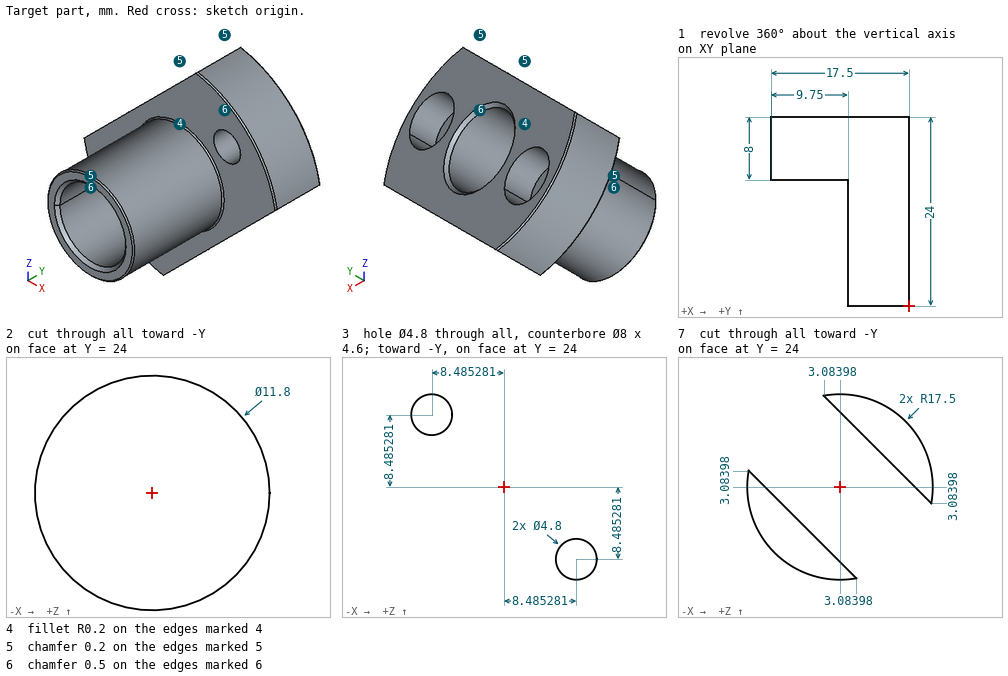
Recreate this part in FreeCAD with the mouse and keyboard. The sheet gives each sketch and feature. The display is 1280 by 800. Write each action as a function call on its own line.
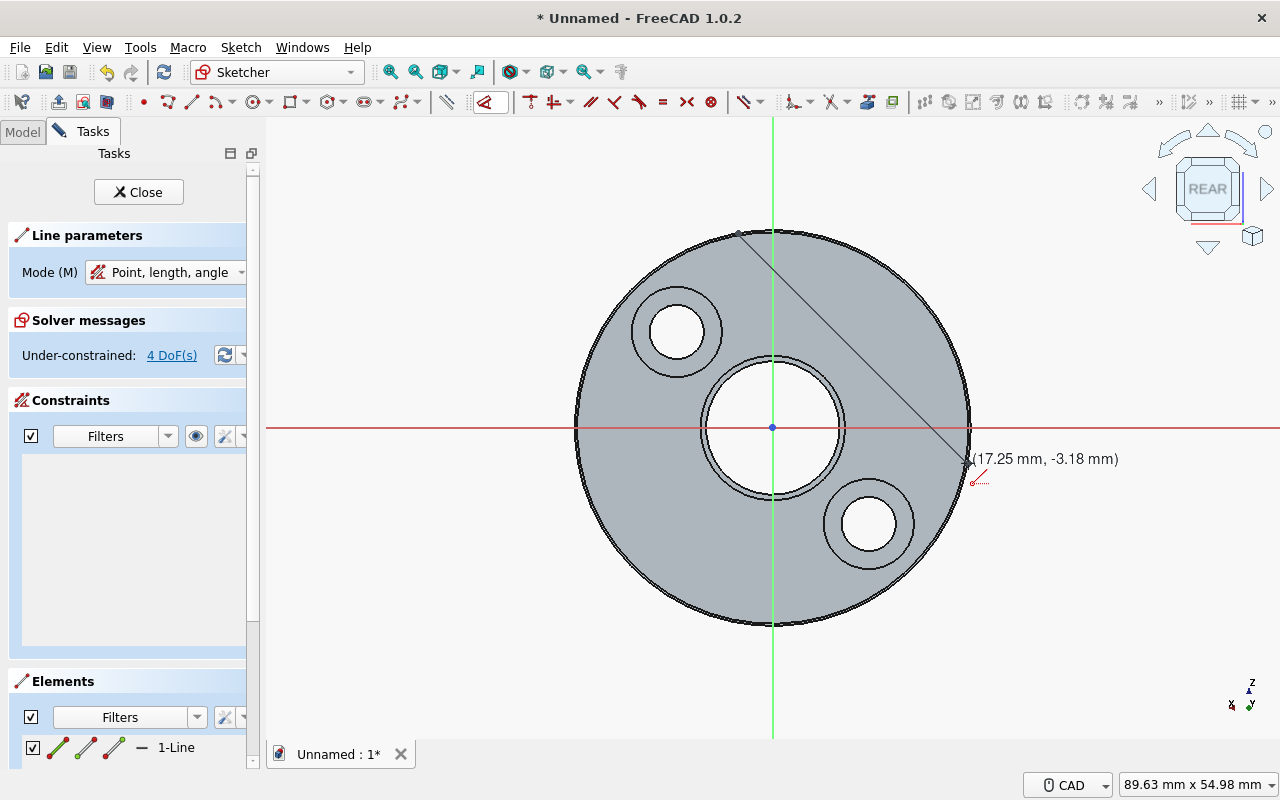
key(g)
key(3)
key(a)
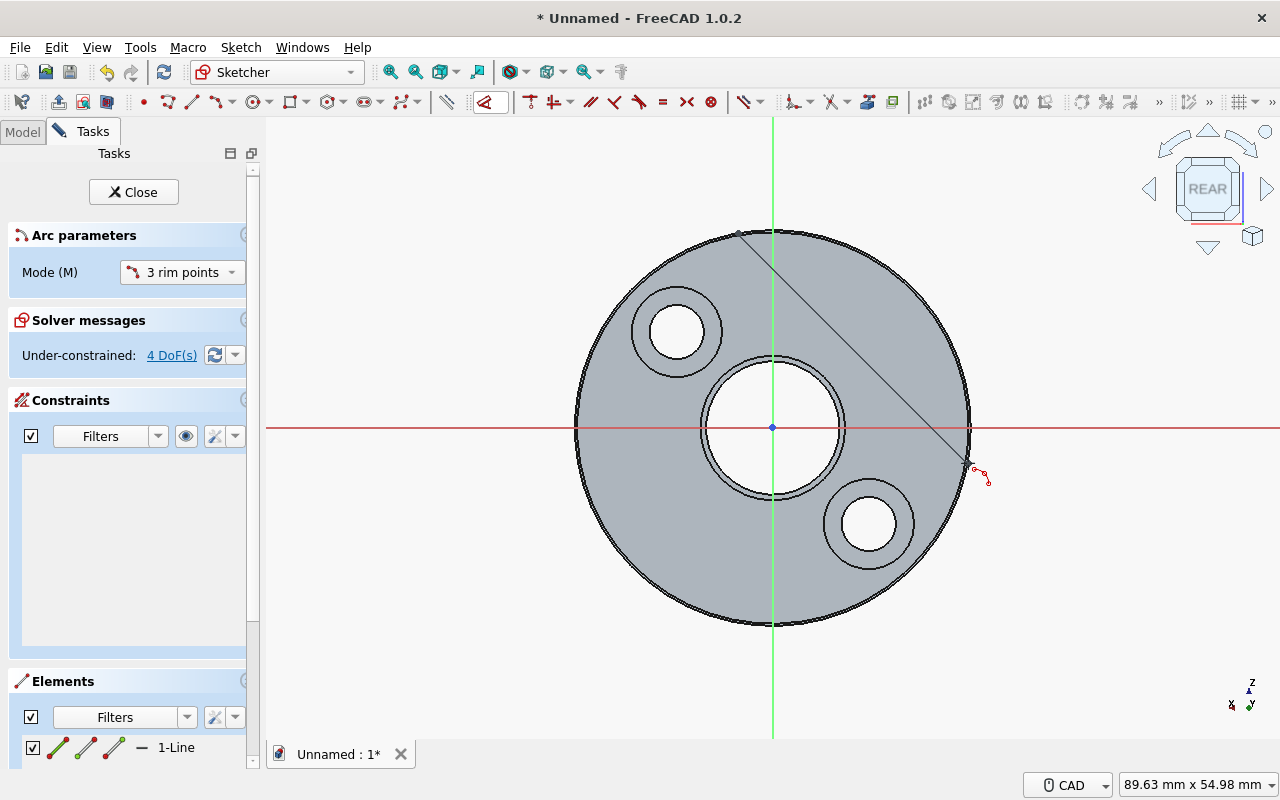
click(968, 464)
click(738, 234)
click(913, 288)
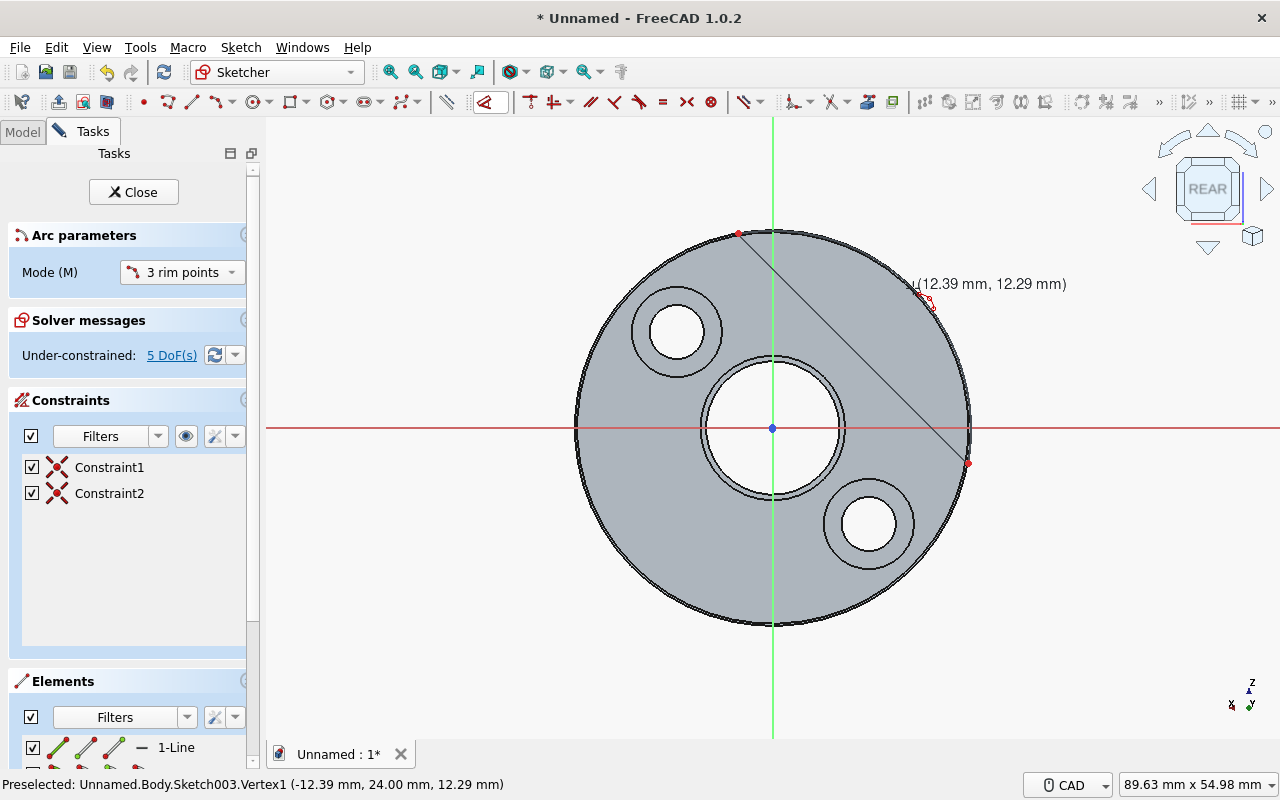
click(192, 102)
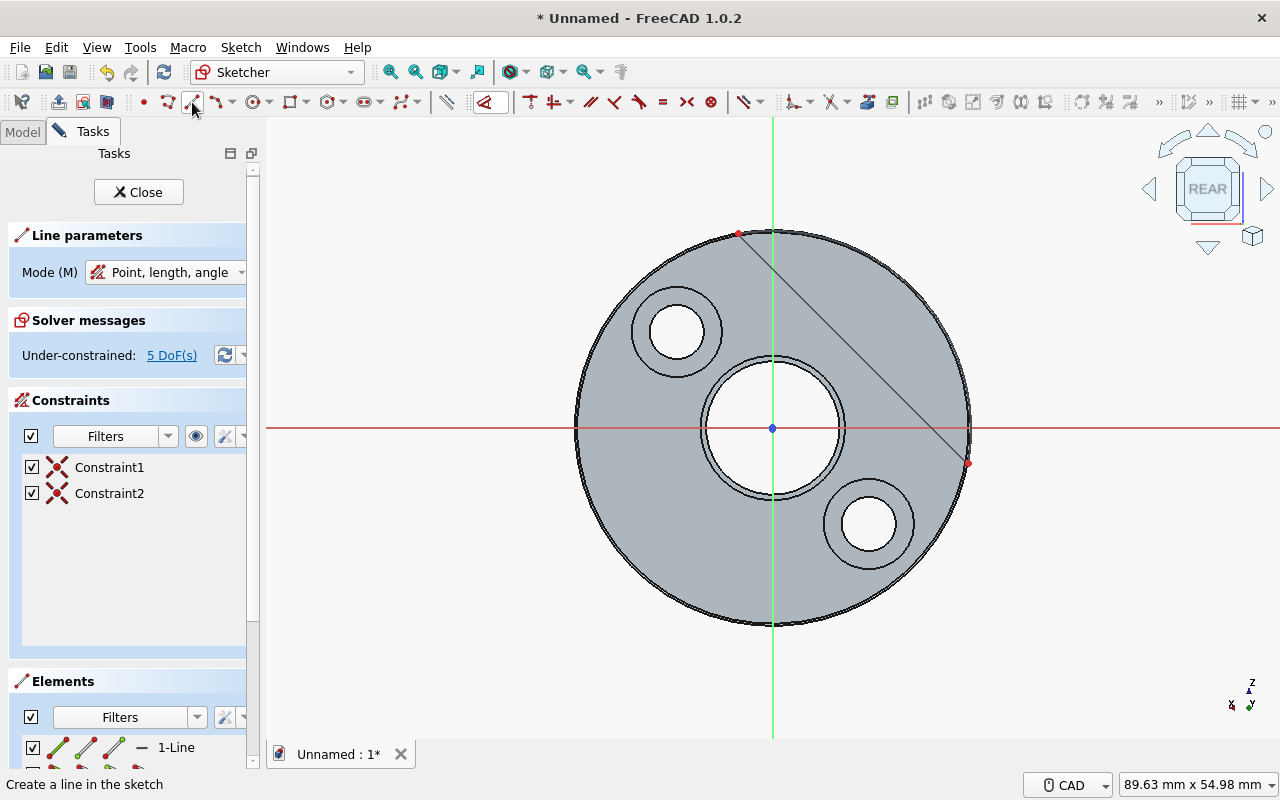
click(808, 623)
click(578, 393)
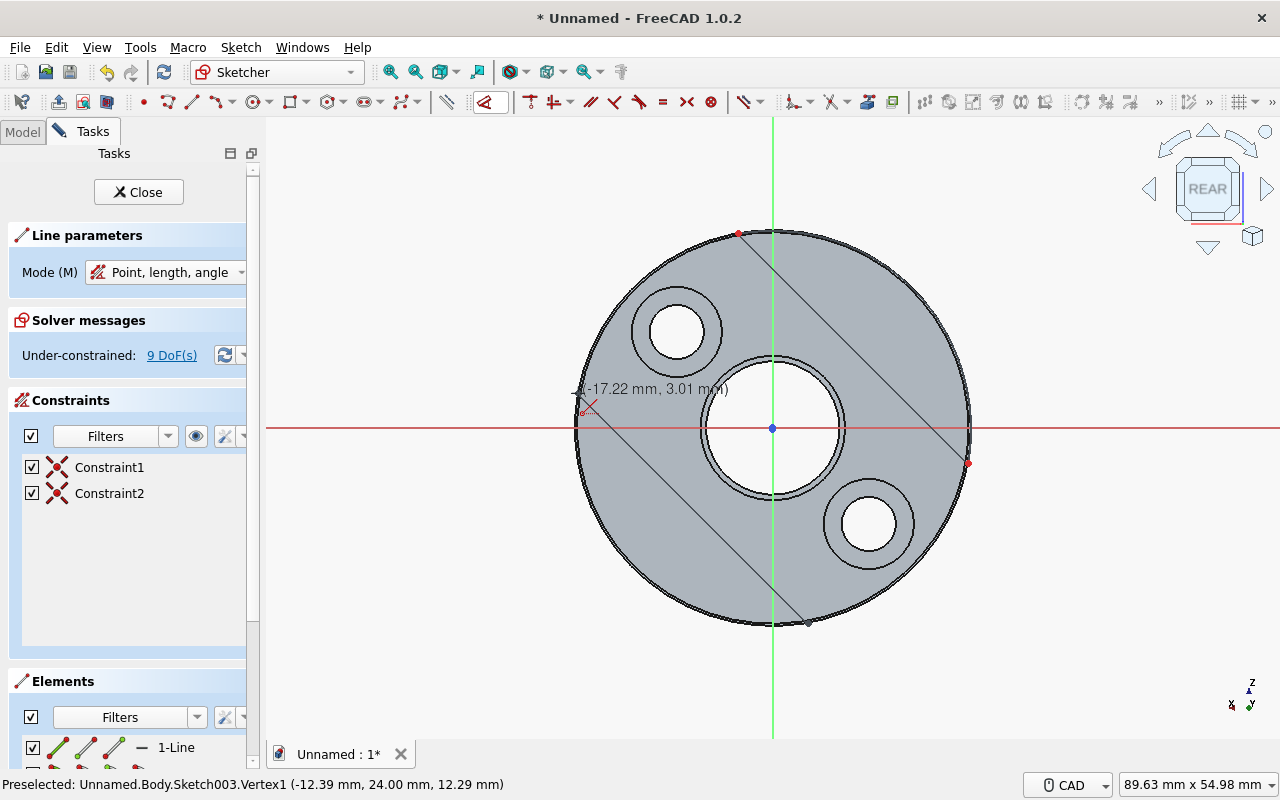
key(g)
key(3)
key(a)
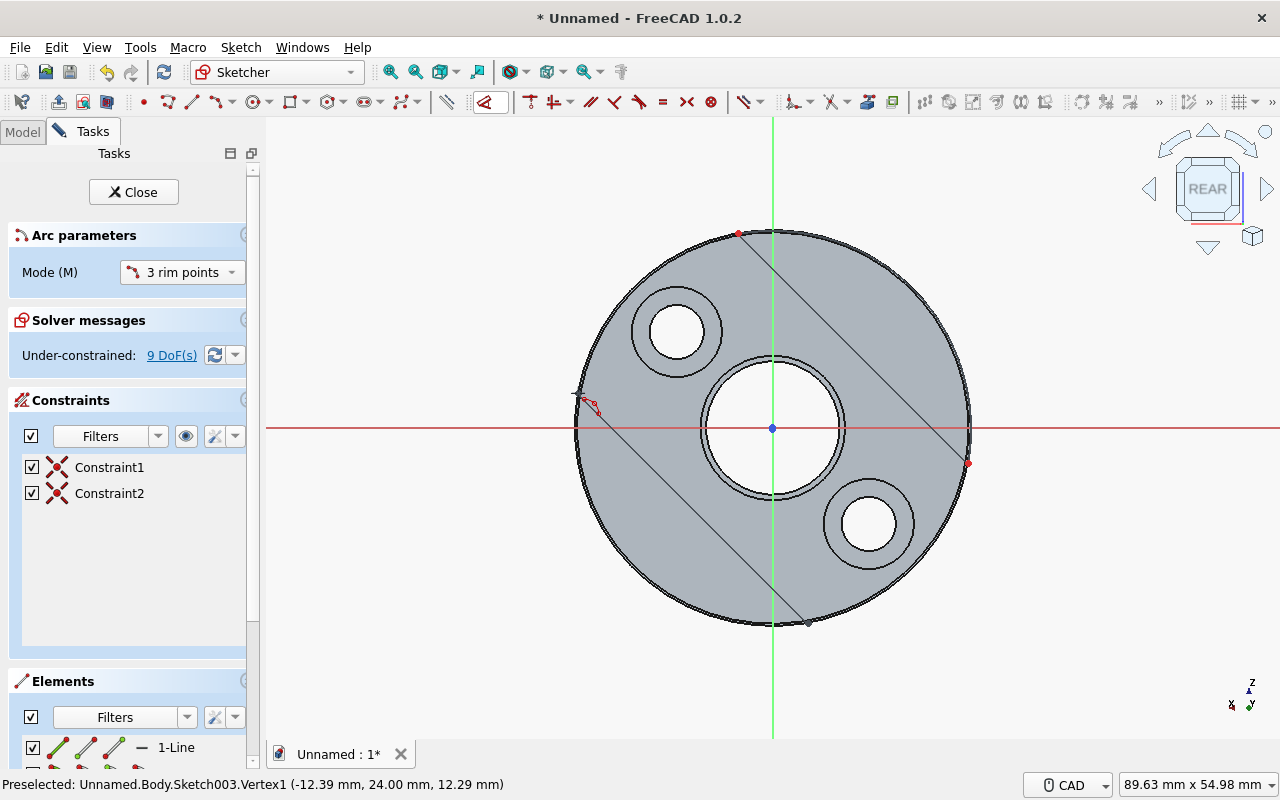
click(578, 394)
click(808, 624)
click(633, 568)
key(Escape)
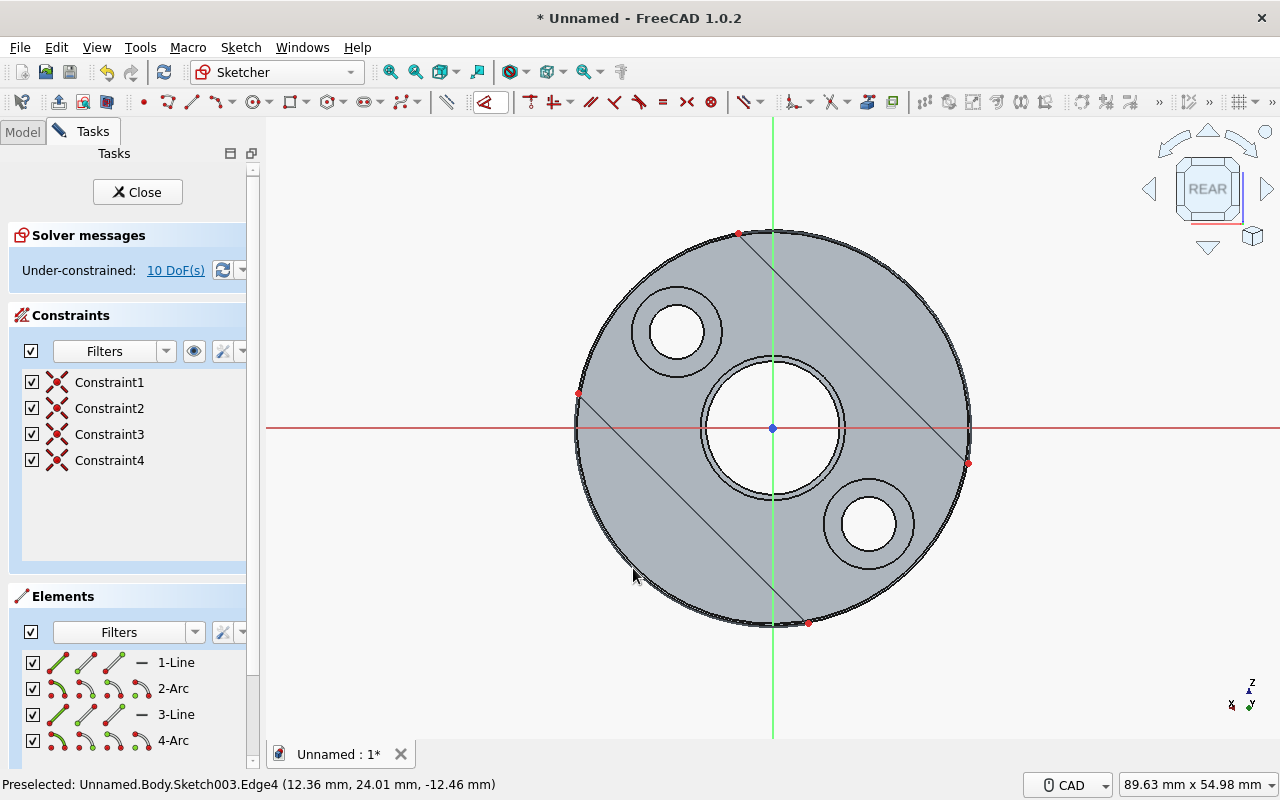
click(955, 352)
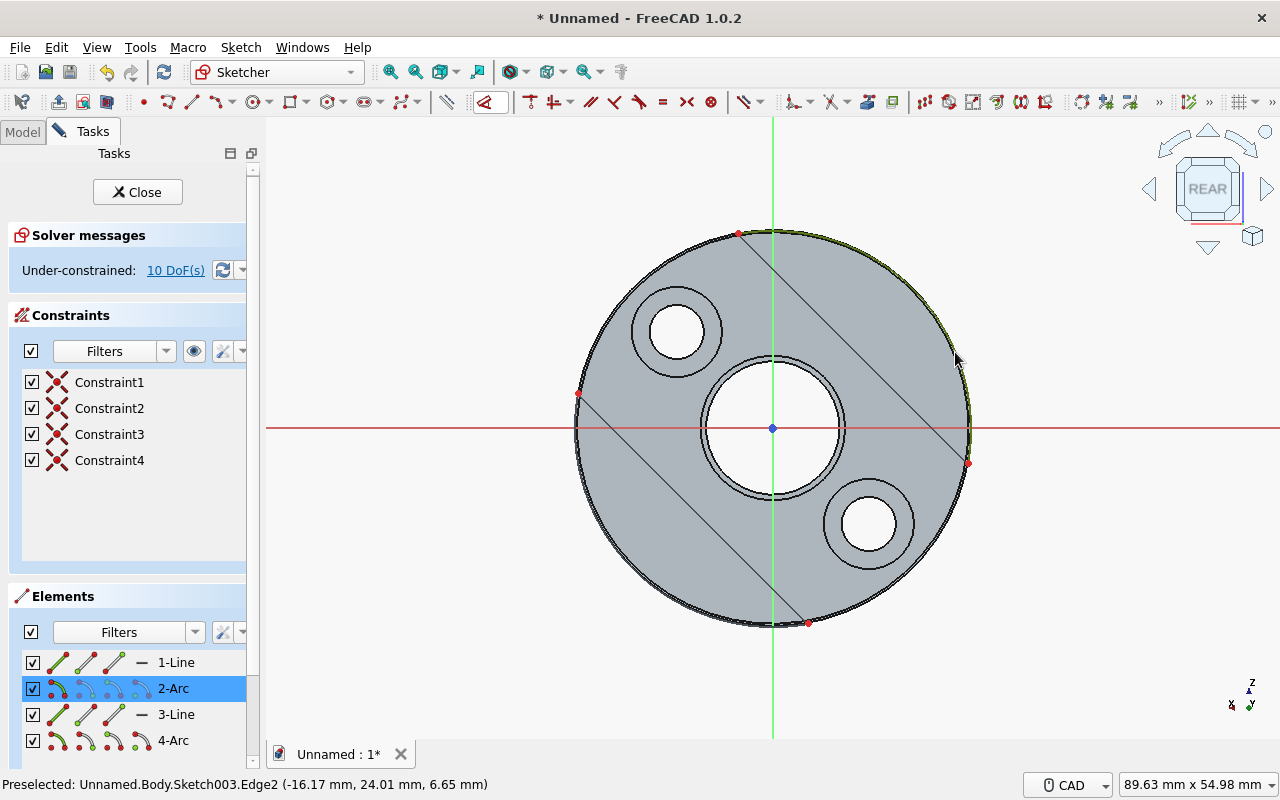
click(591, 506)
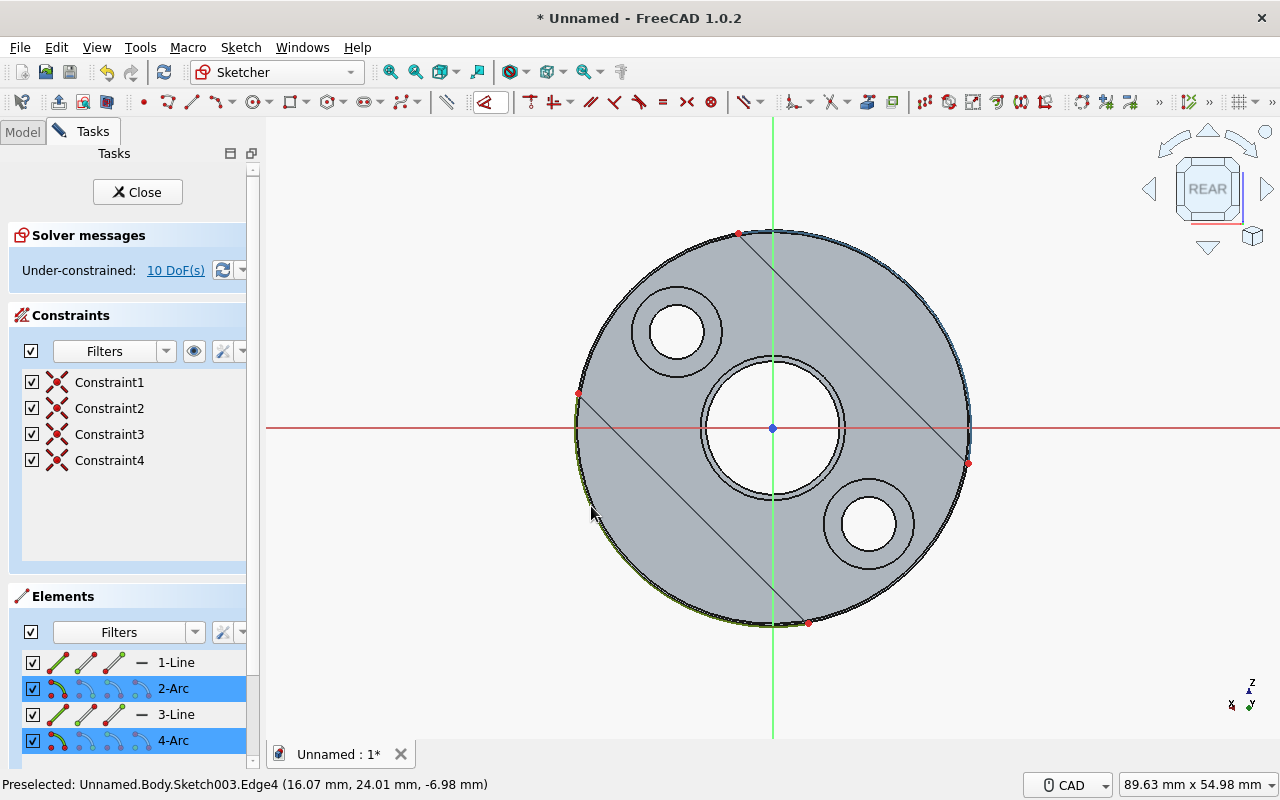
key(c)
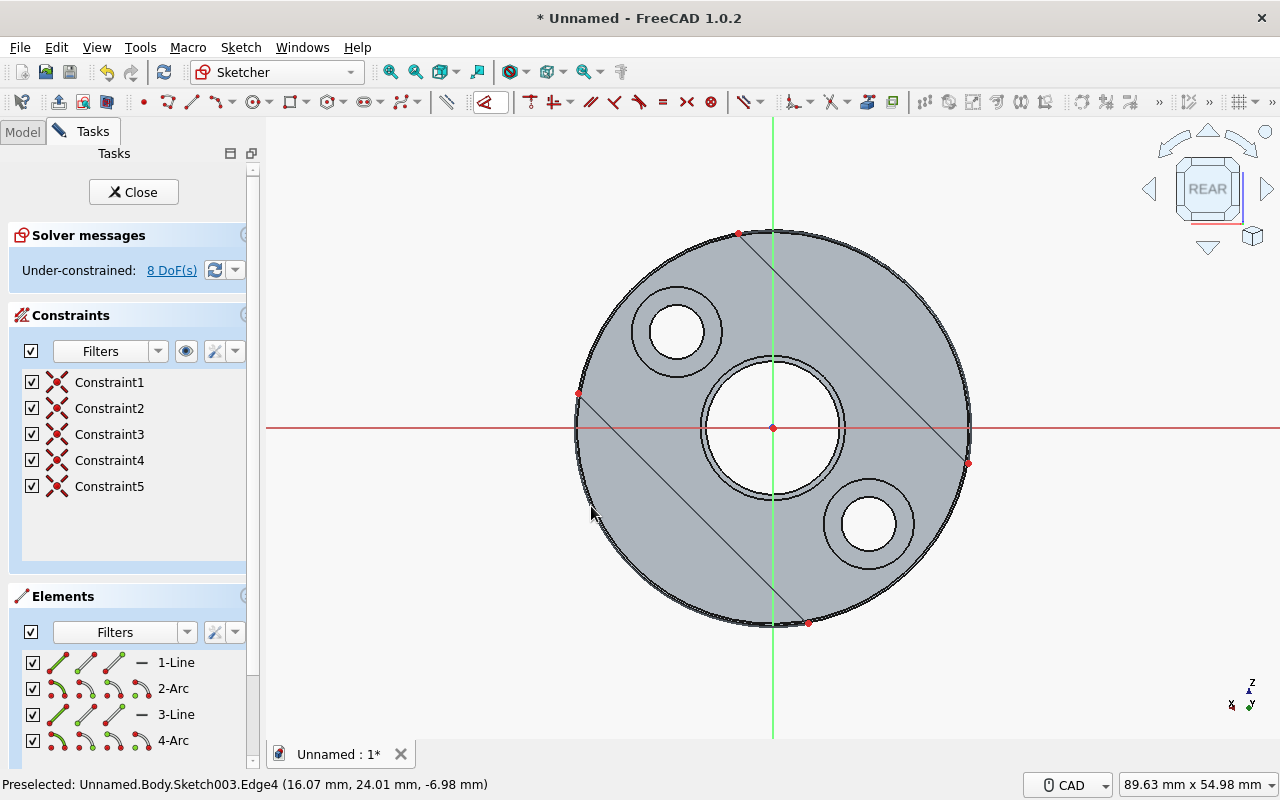
drag(763, 418, 783, 439)